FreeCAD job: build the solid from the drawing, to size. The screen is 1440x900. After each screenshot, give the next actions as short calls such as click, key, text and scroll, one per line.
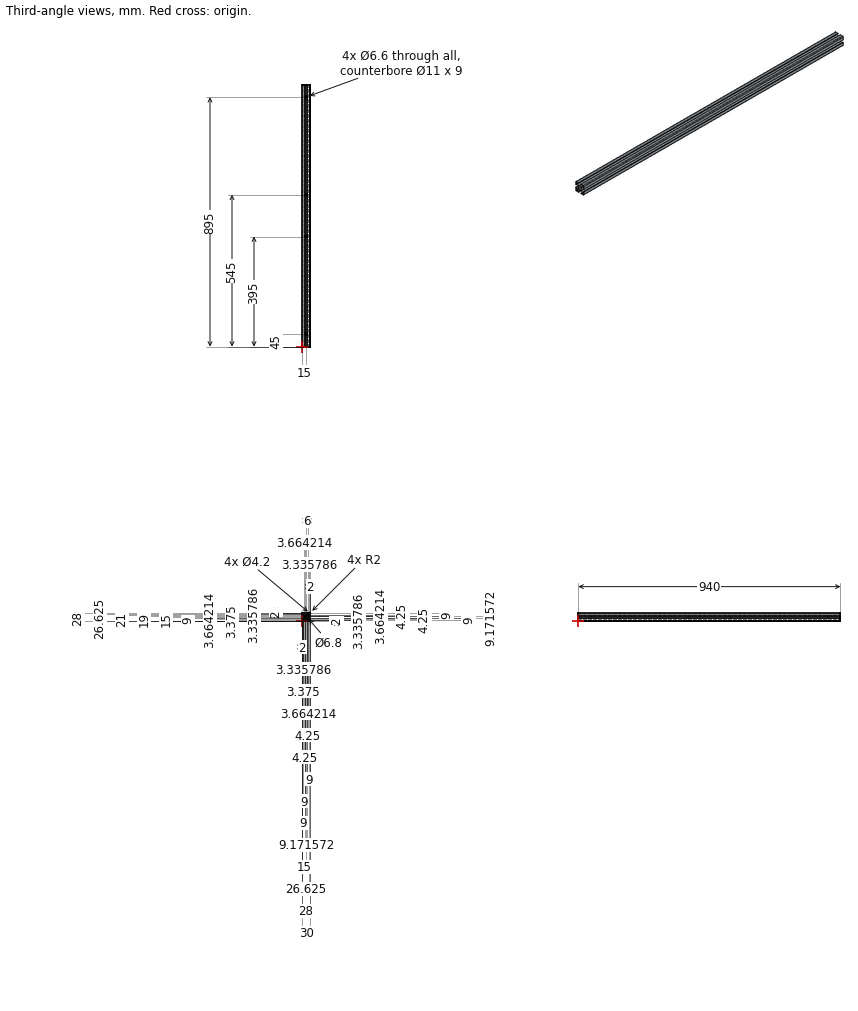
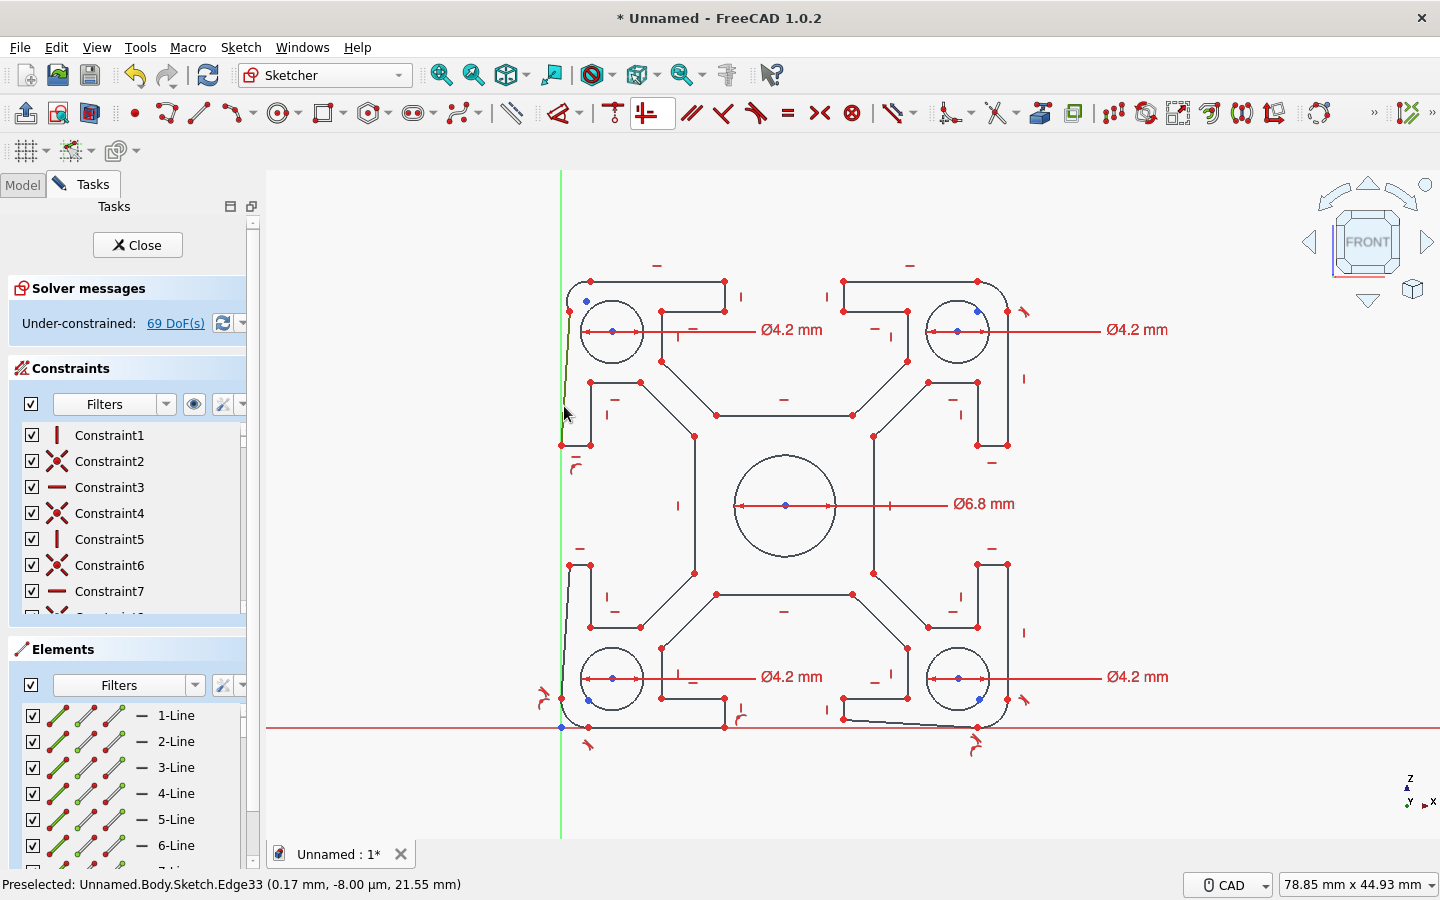
click(577, 284)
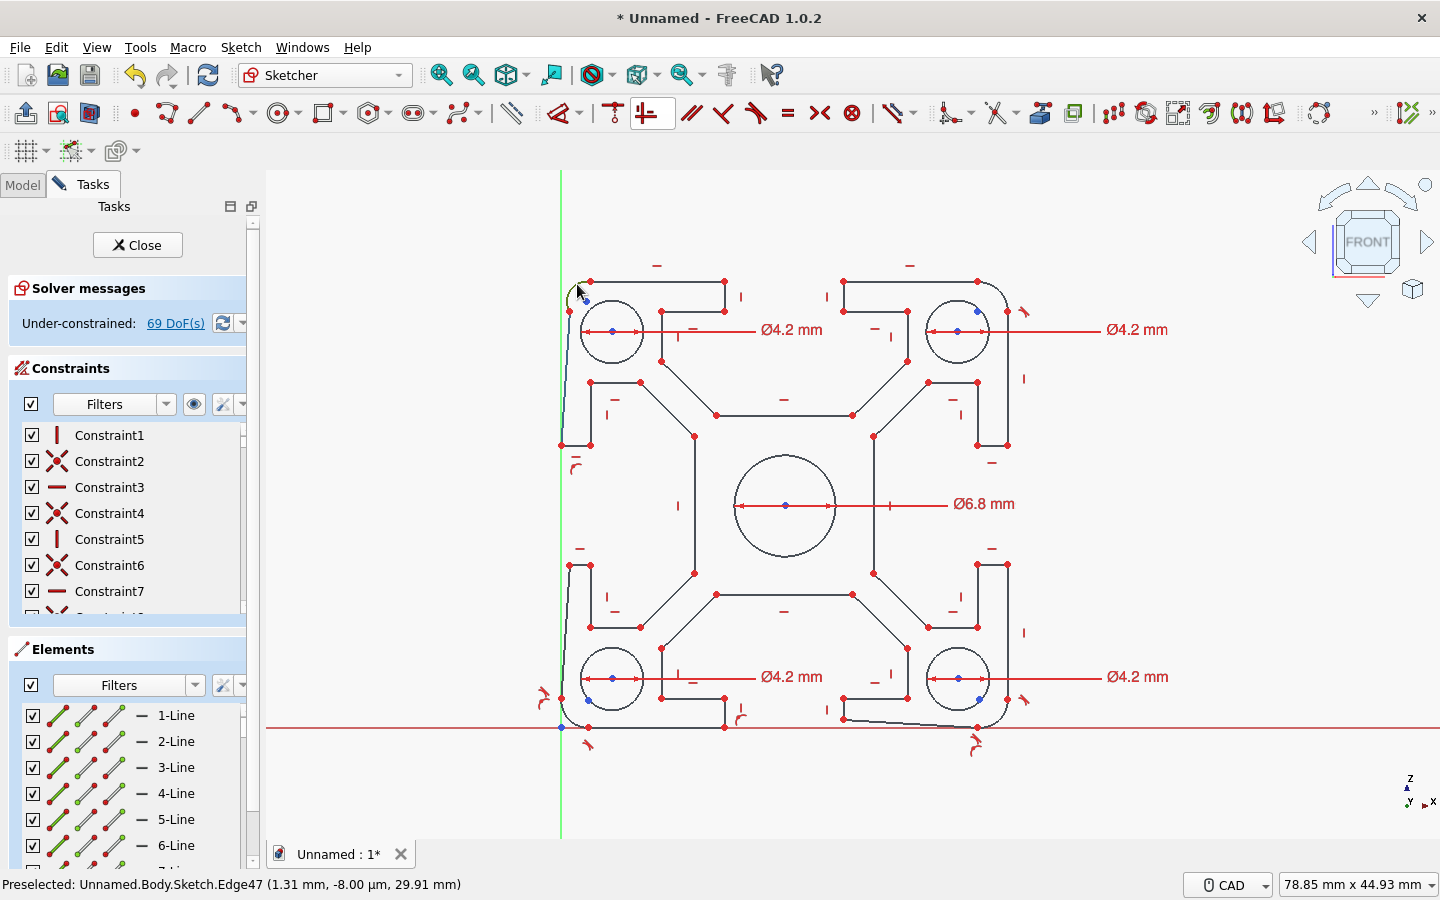
click(756, 114)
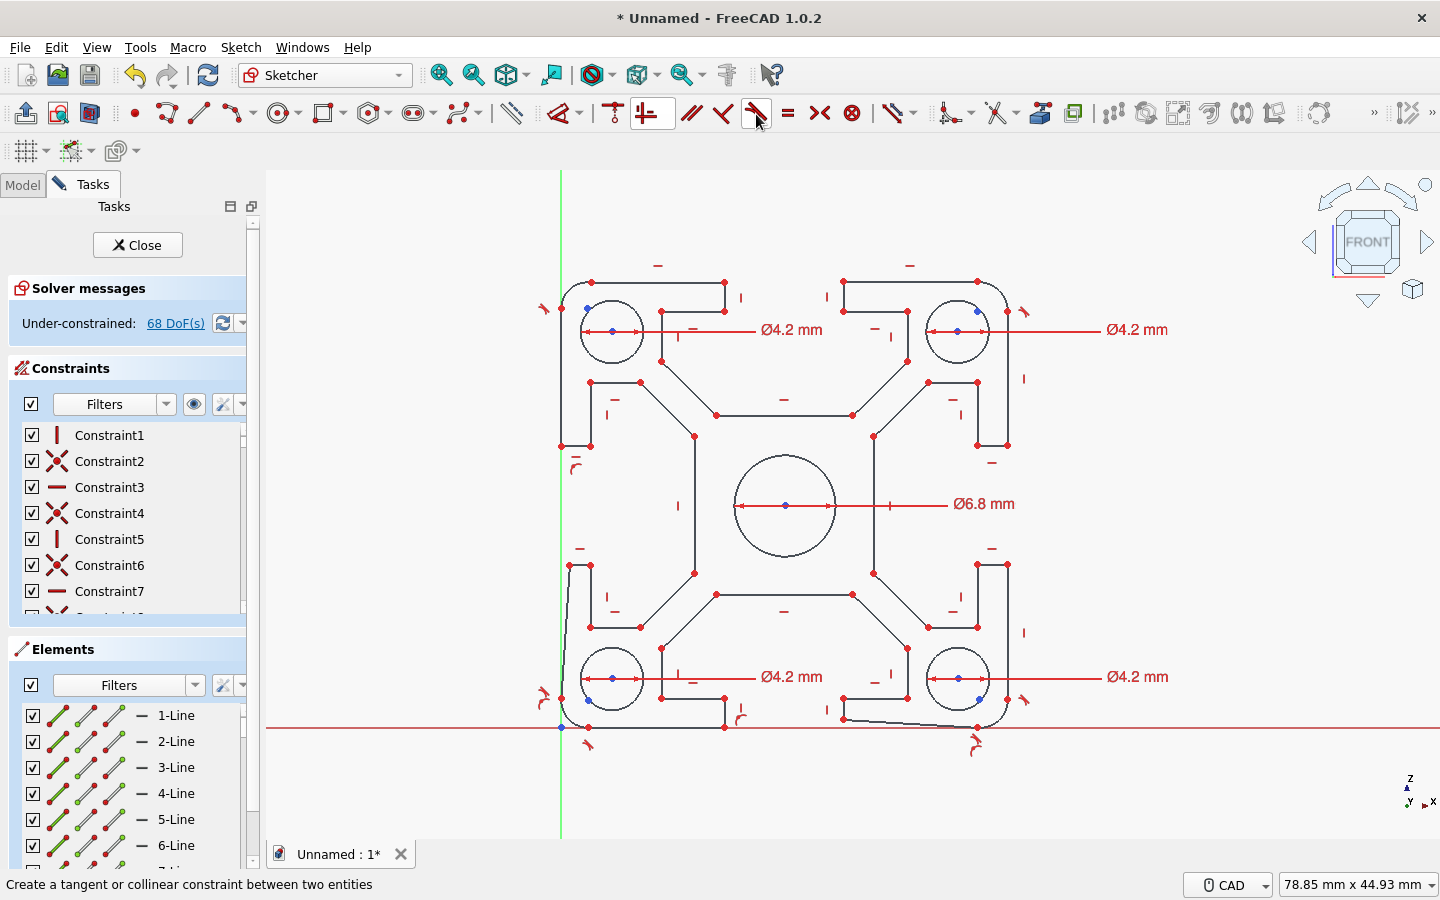
click(631, 283)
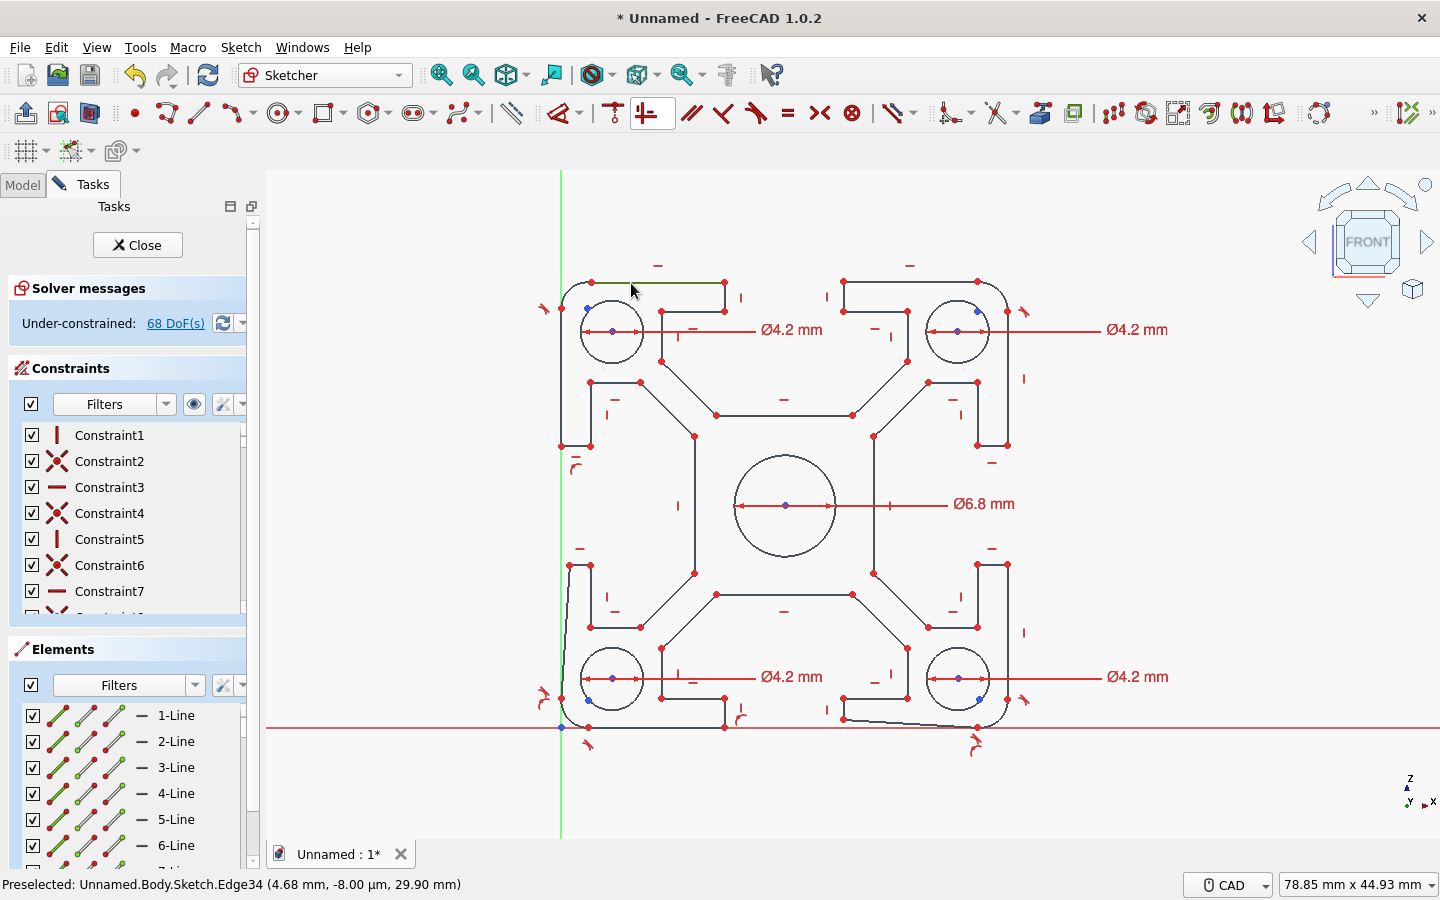
click(578, 284)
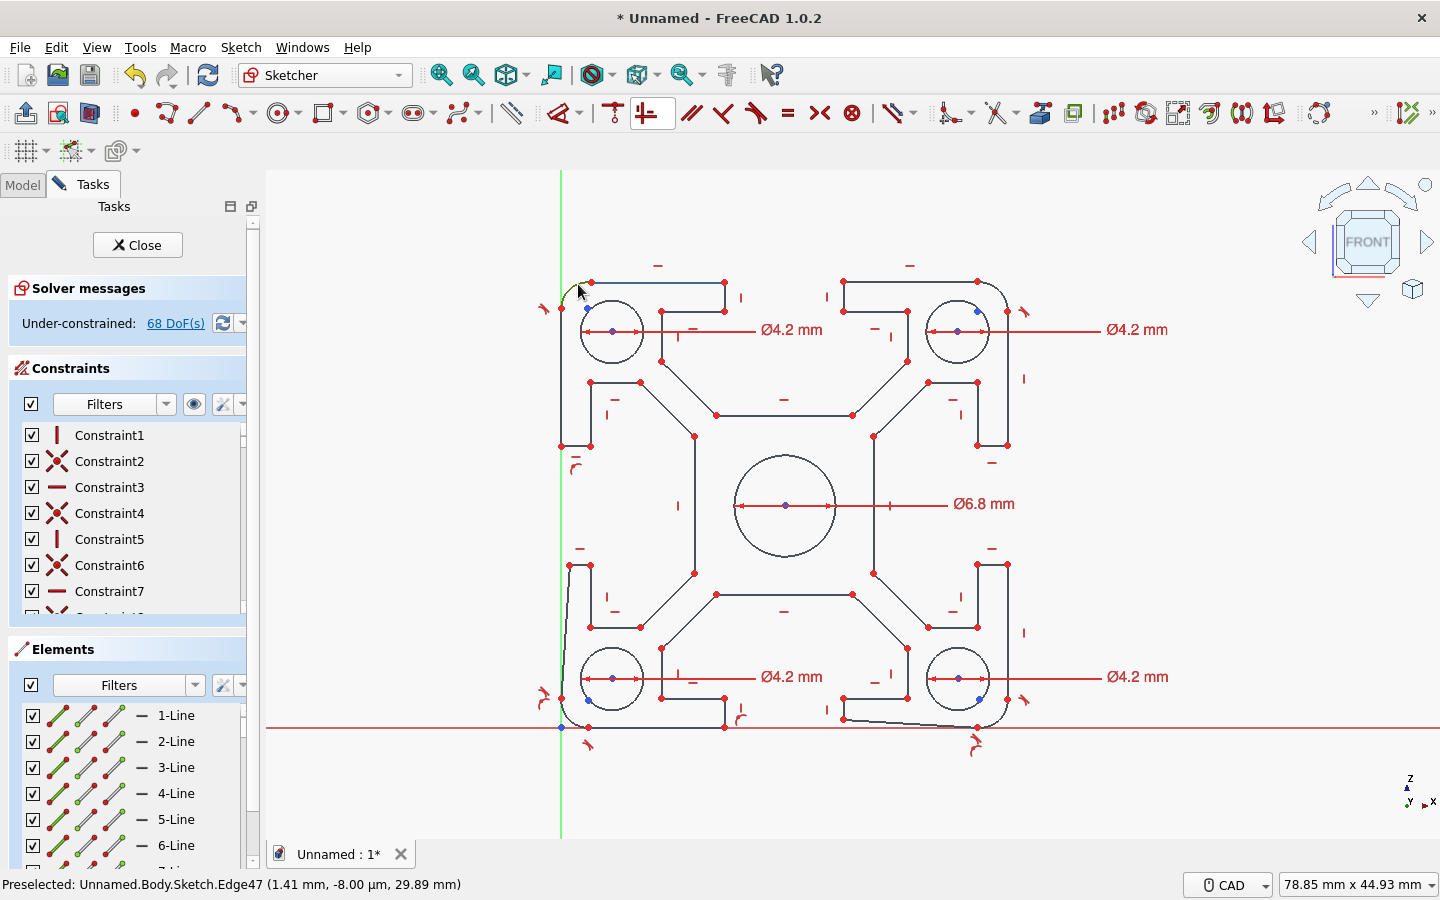
click(756, 114)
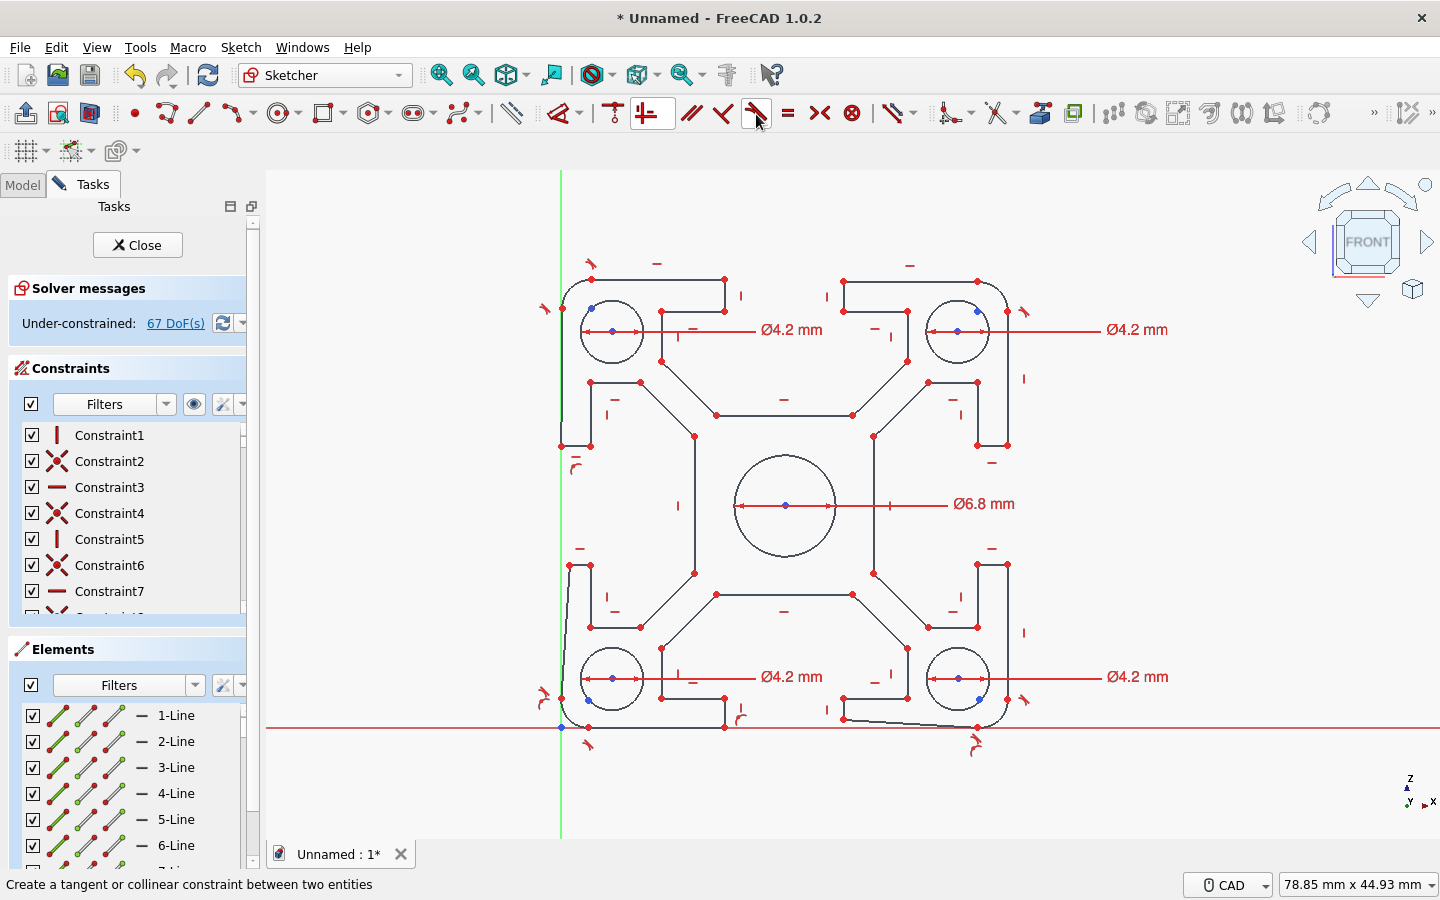
click(884, 282)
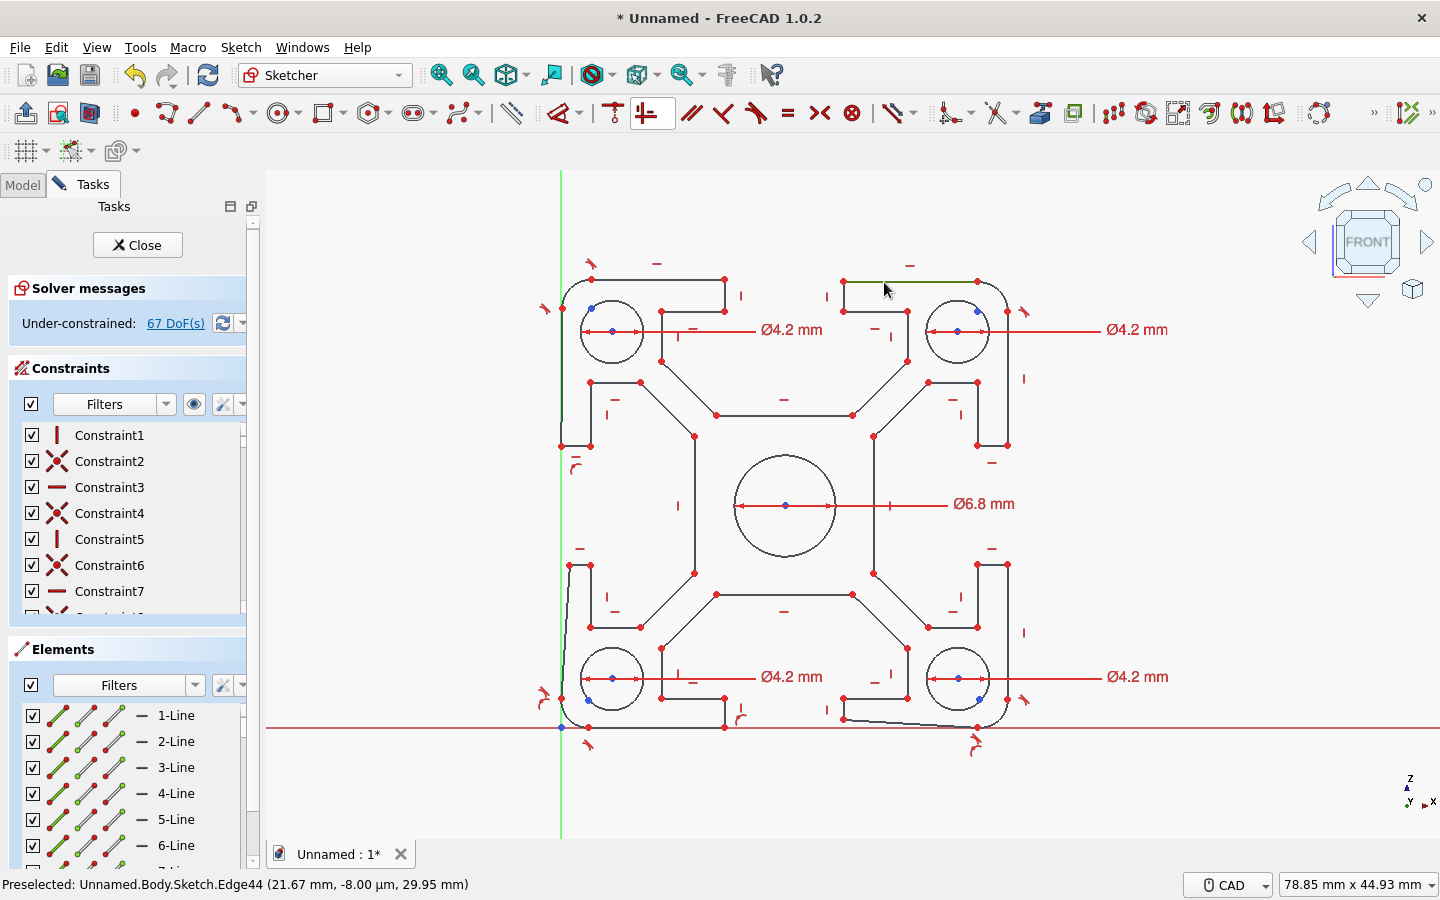
click(1005, 298)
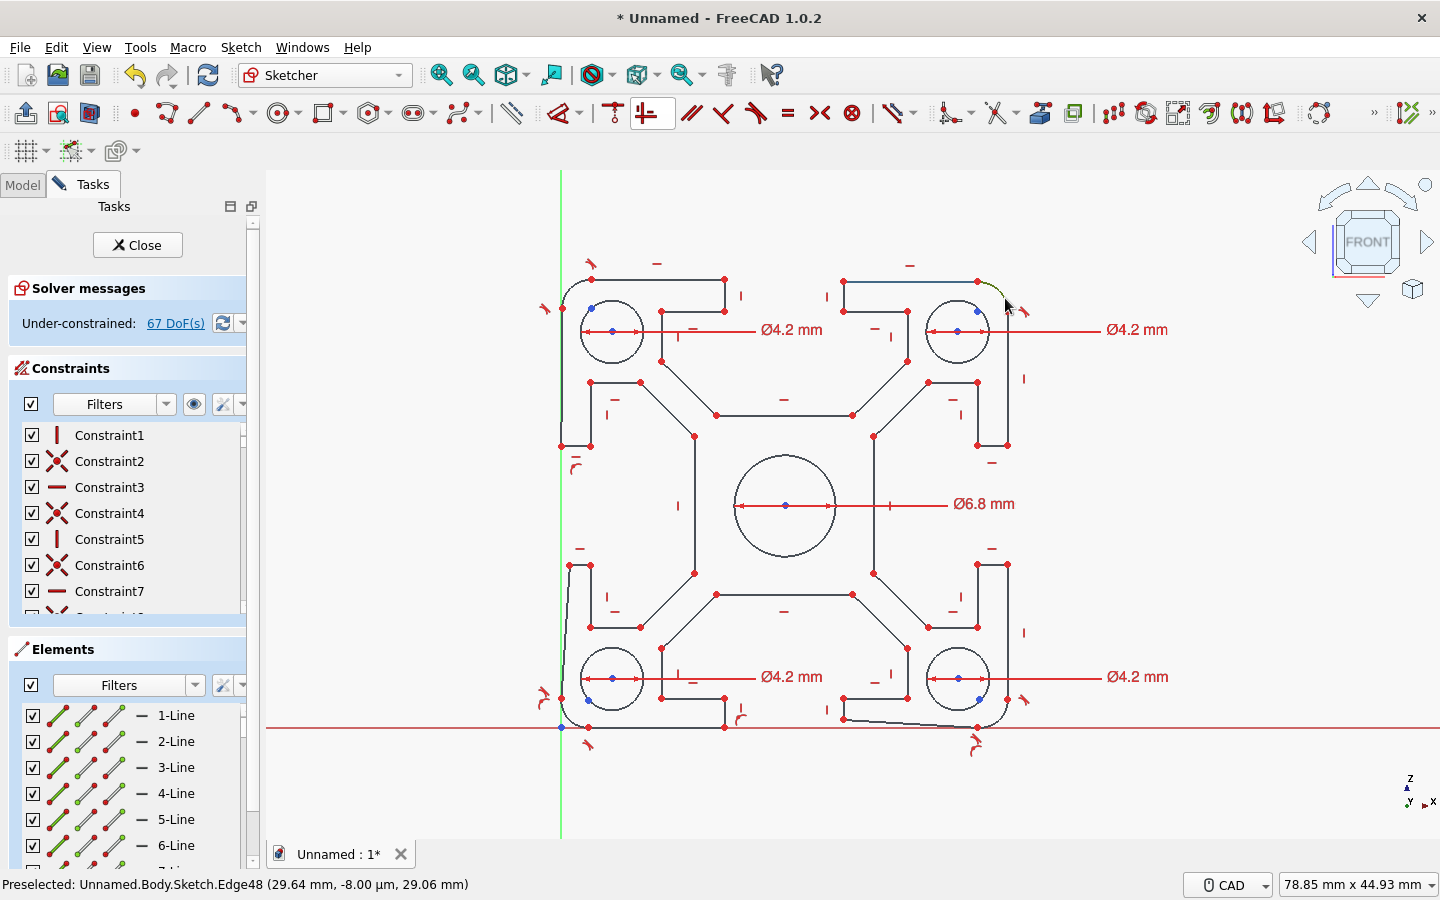
click(756, 114)